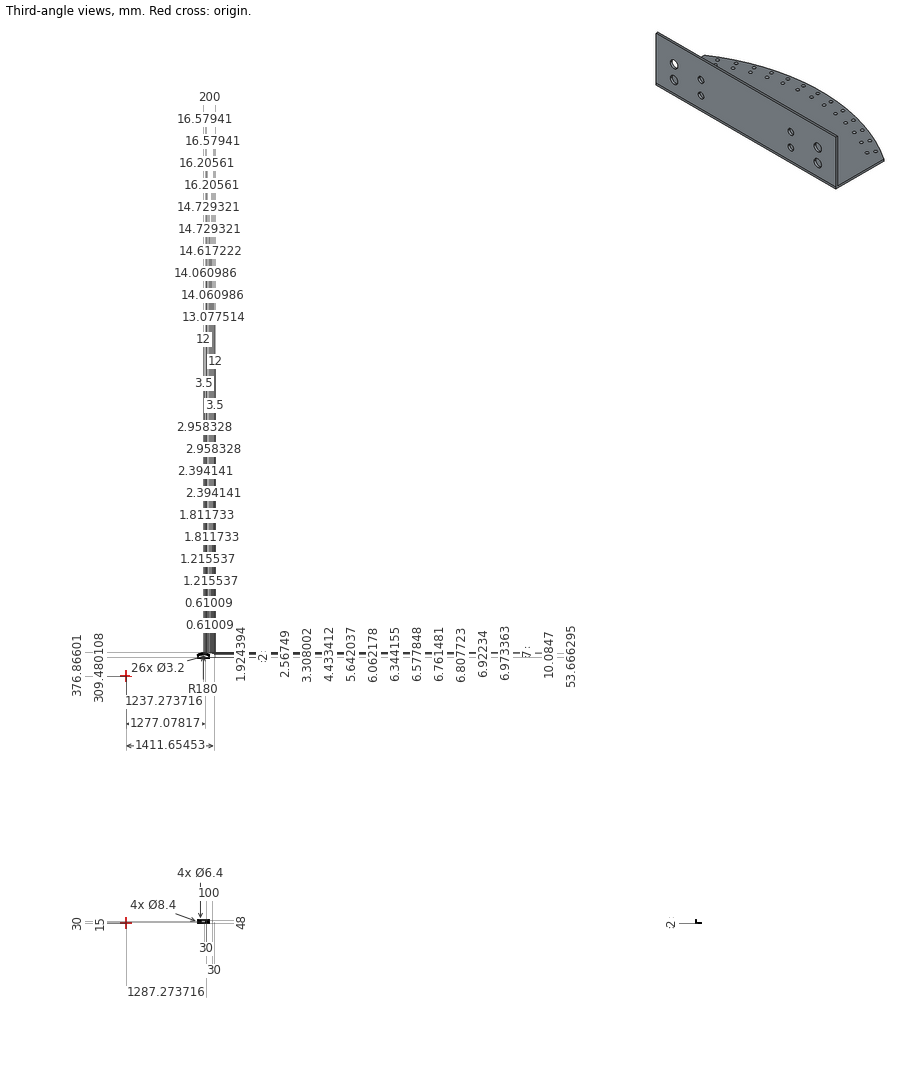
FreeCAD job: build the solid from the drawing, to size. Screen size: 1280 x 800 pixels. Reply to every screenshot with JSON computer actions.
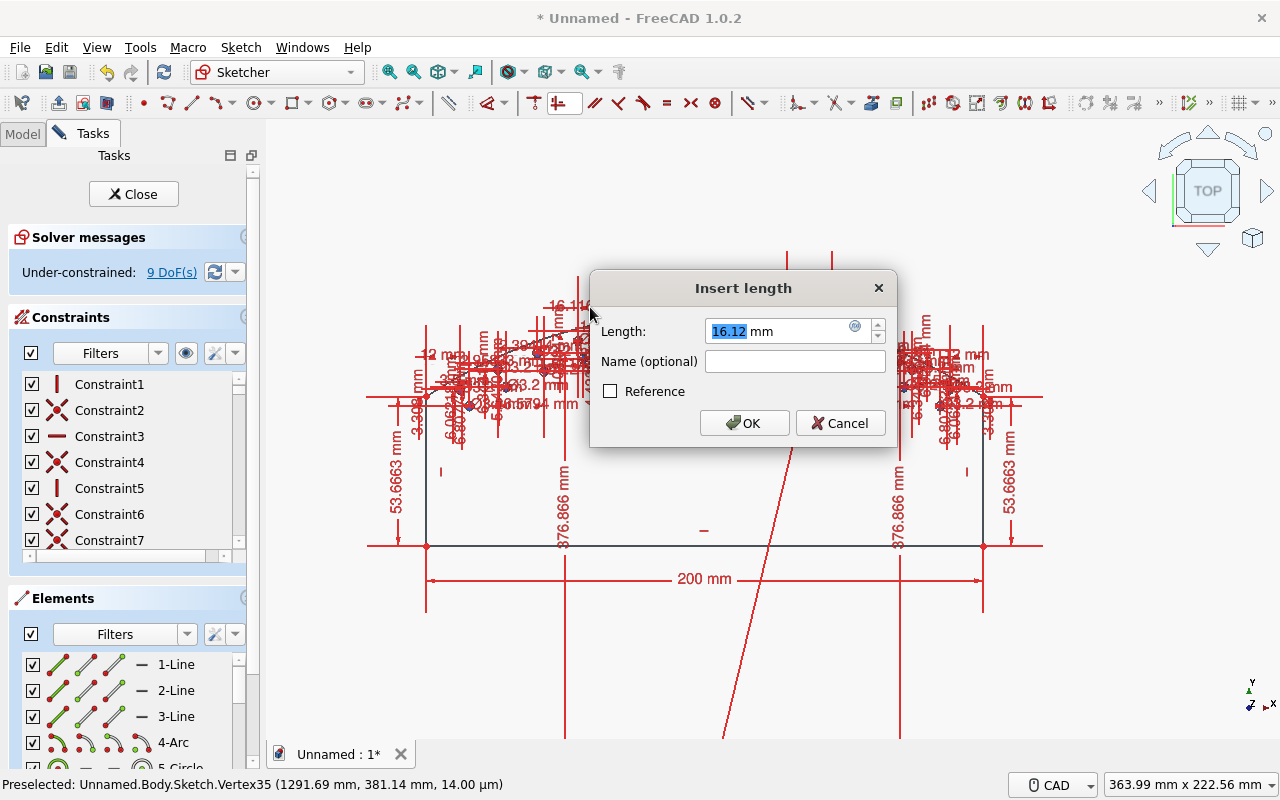
{"action": "type", "text": "16.20561"}
{"action": "key", "text": "Return"}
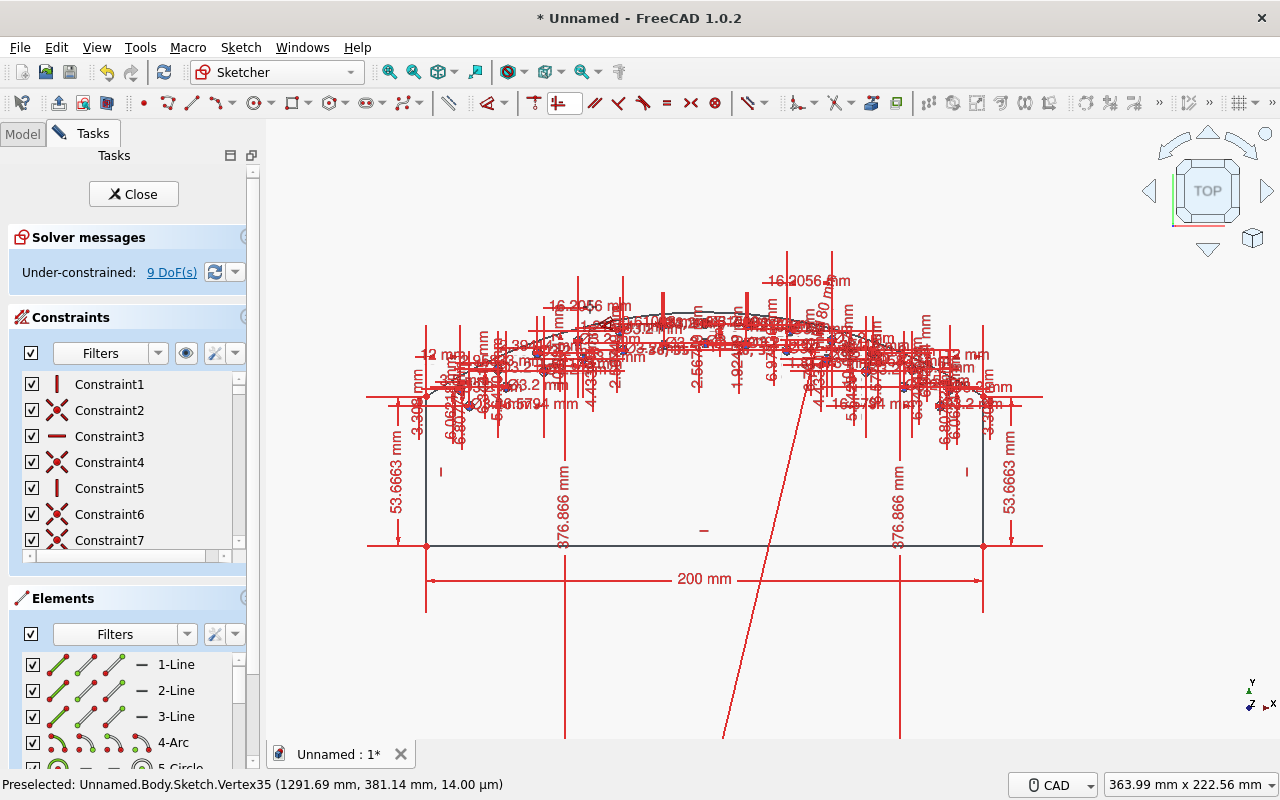
{"action": "scroll", "coordinate": [583, 359], "scroll_direction": "up", "scroll_amount": 4}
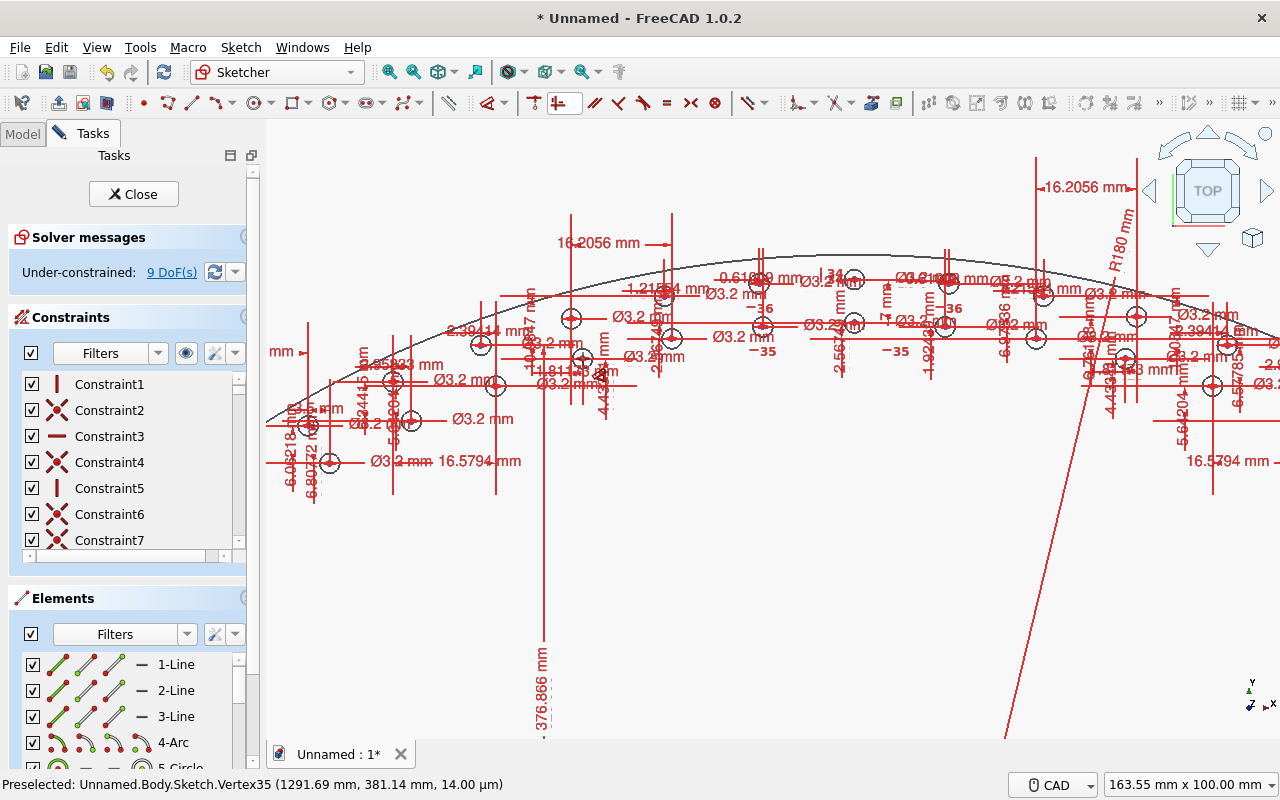
{"action": "left_click", "coordinate": [583, 359]}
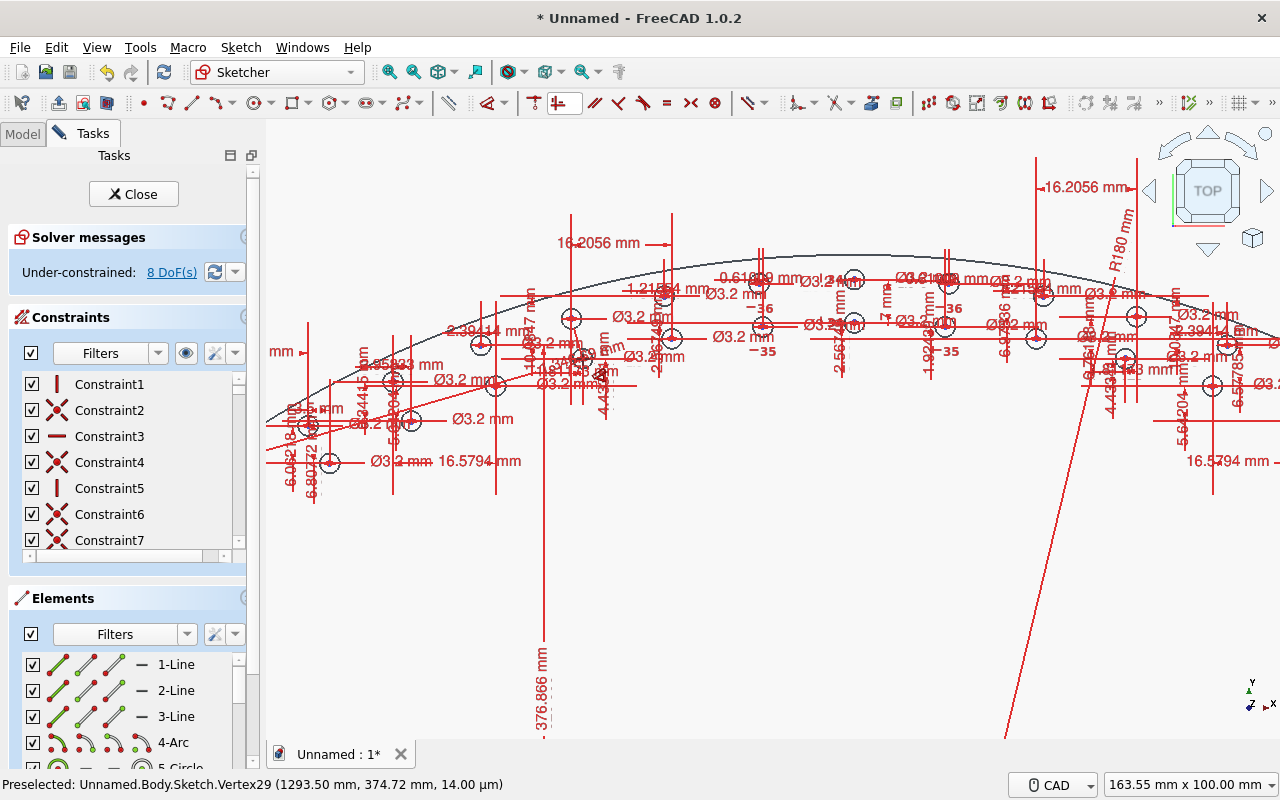
{"action": "left_click", "coordinate": [571, 319]}
{"action": "left_click", "coordinate": [417, 325]}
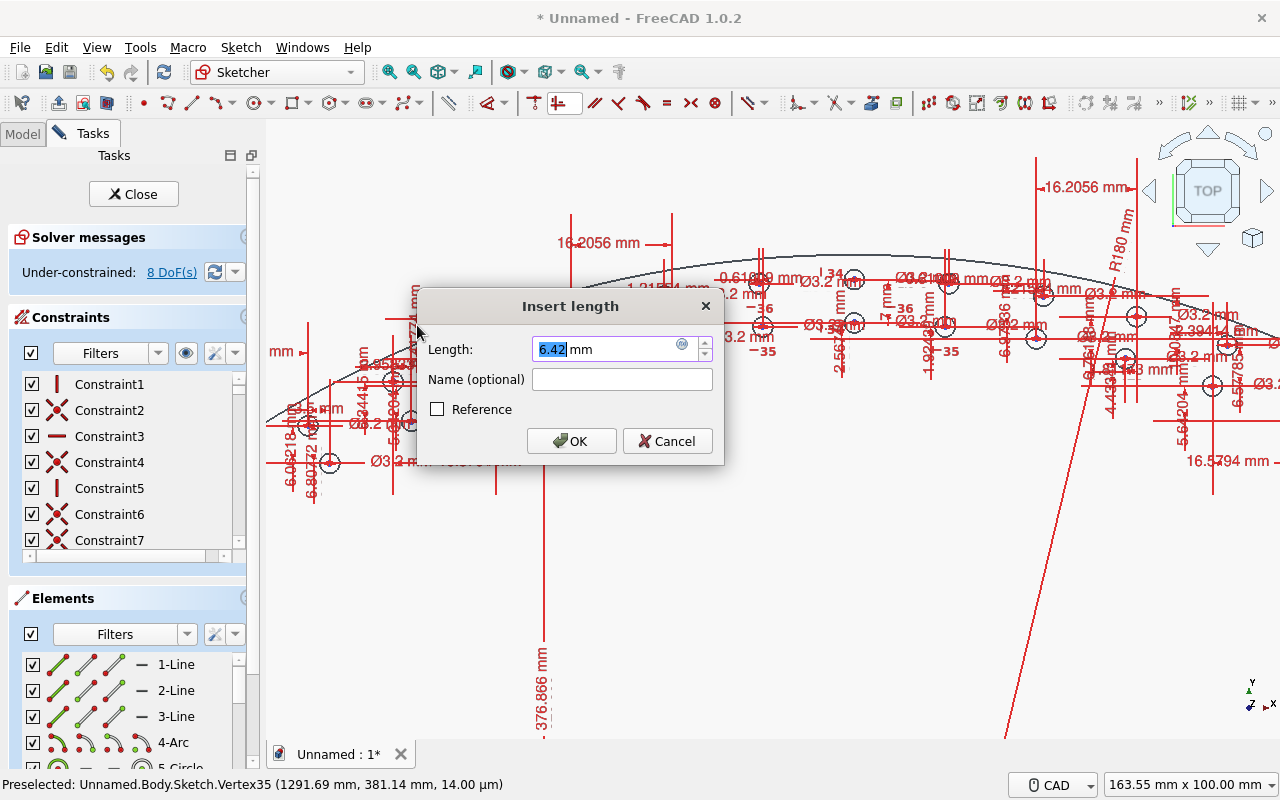
{"action": "type", "text": "6.761481"}
{"action": "key", "text": "Return"}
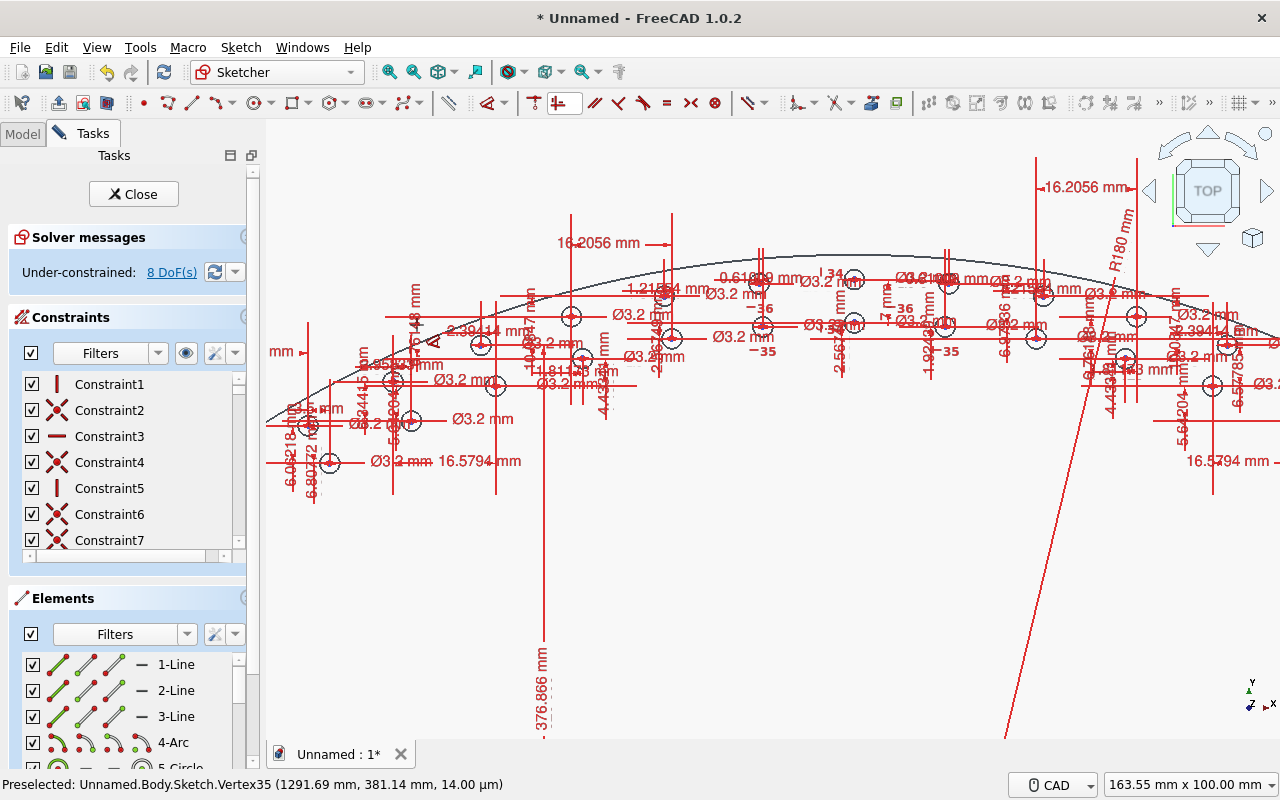
{"action": "scroll", "coordinate": [582, 359], "scroll_direction": "down", "scroll_amount": 4}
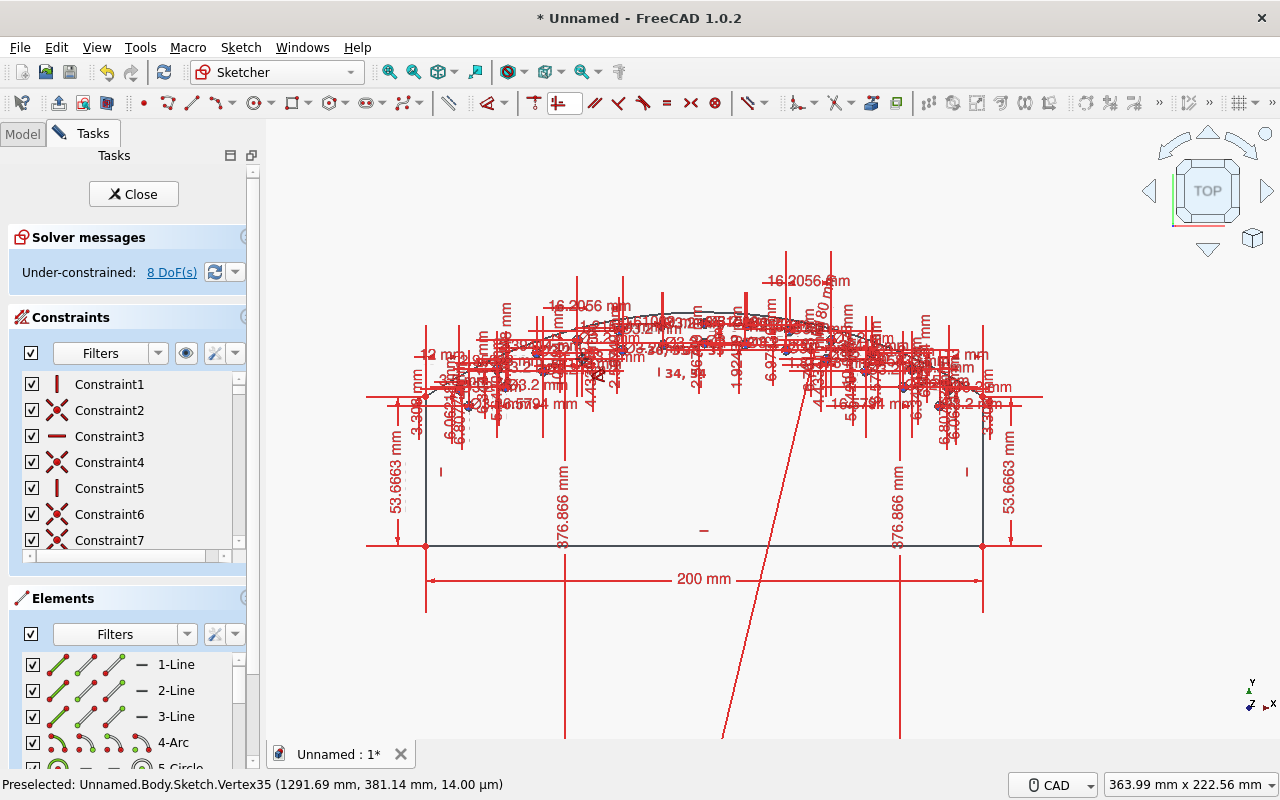
{"action": "left_click", "coordinate": [912, 369]}
{"action": "left_click", "coordinate": [387, 335]}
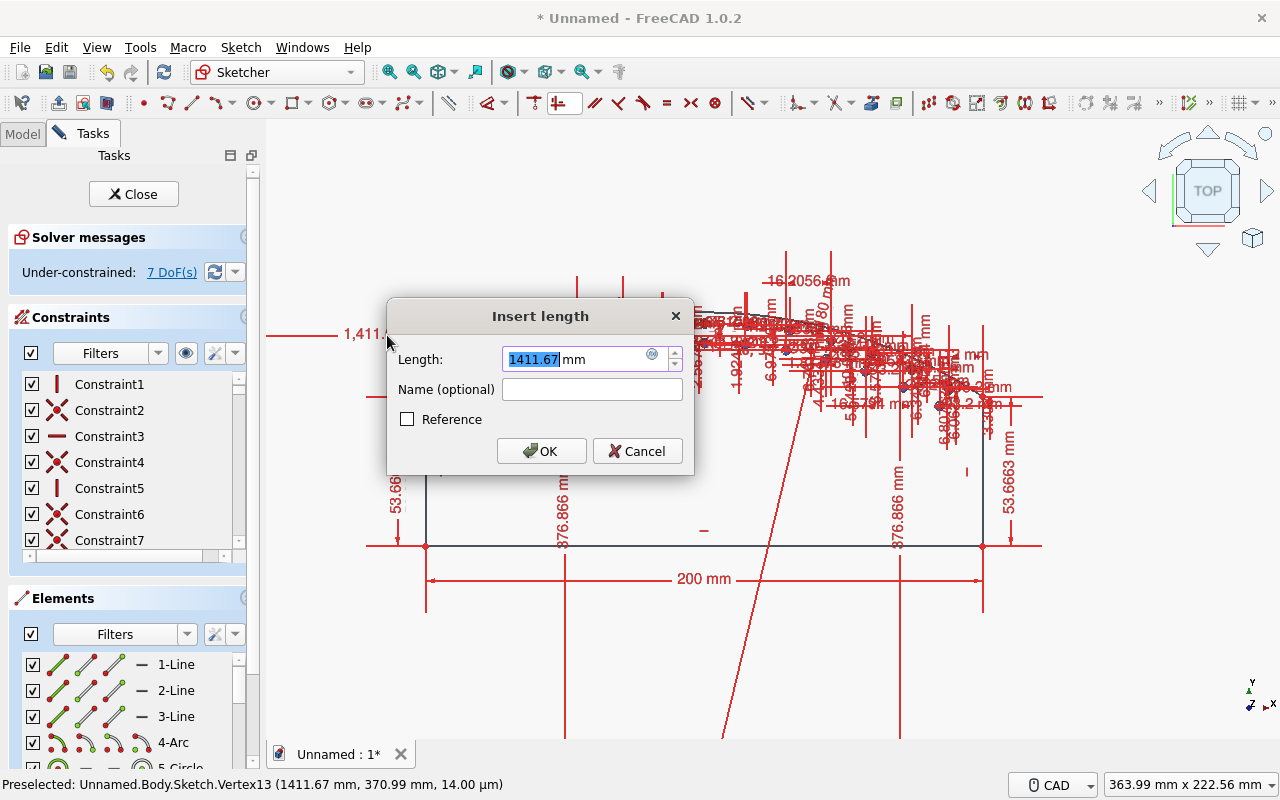
{"action": "type", "text": "1411.65453"}
{"action": "key", "text": "Return"}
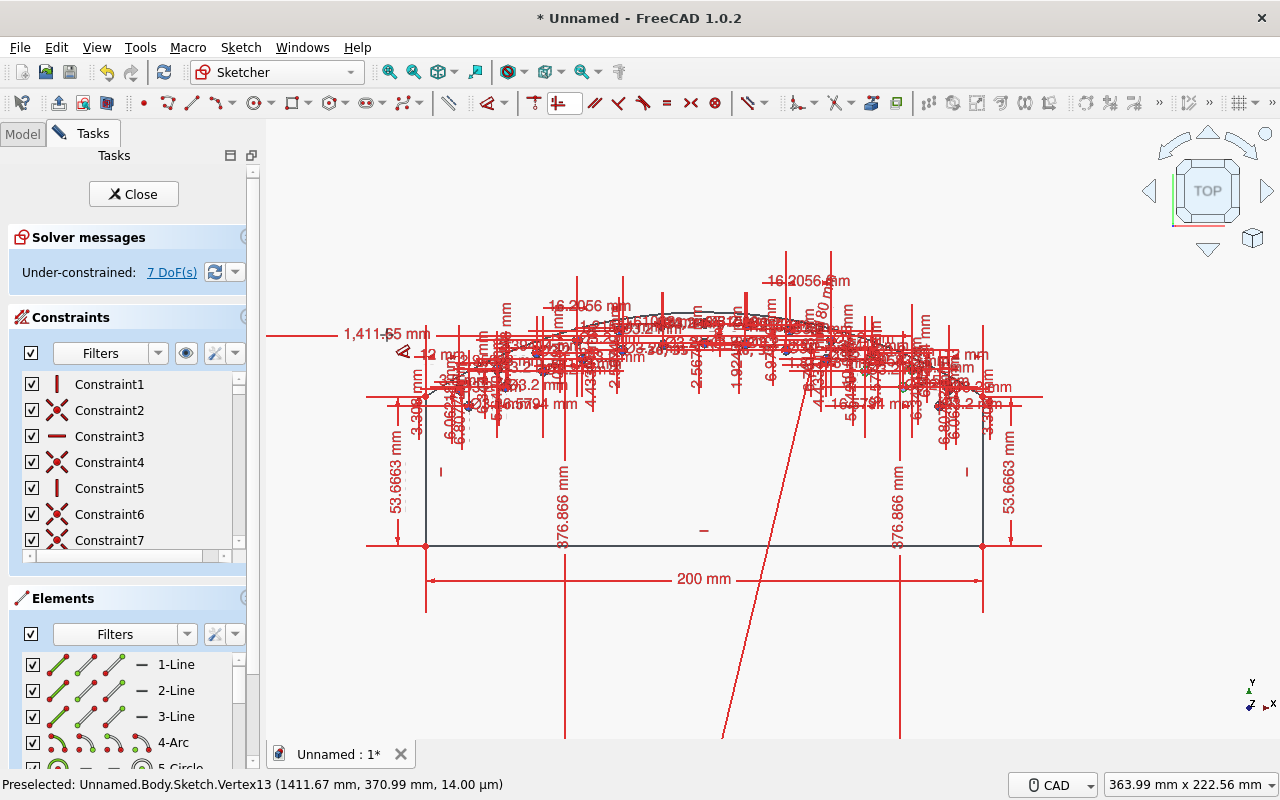
{"action": "left_click", "coordinate": [537, 353]}
{"action": "left_click", "coordinate": [471, 319]}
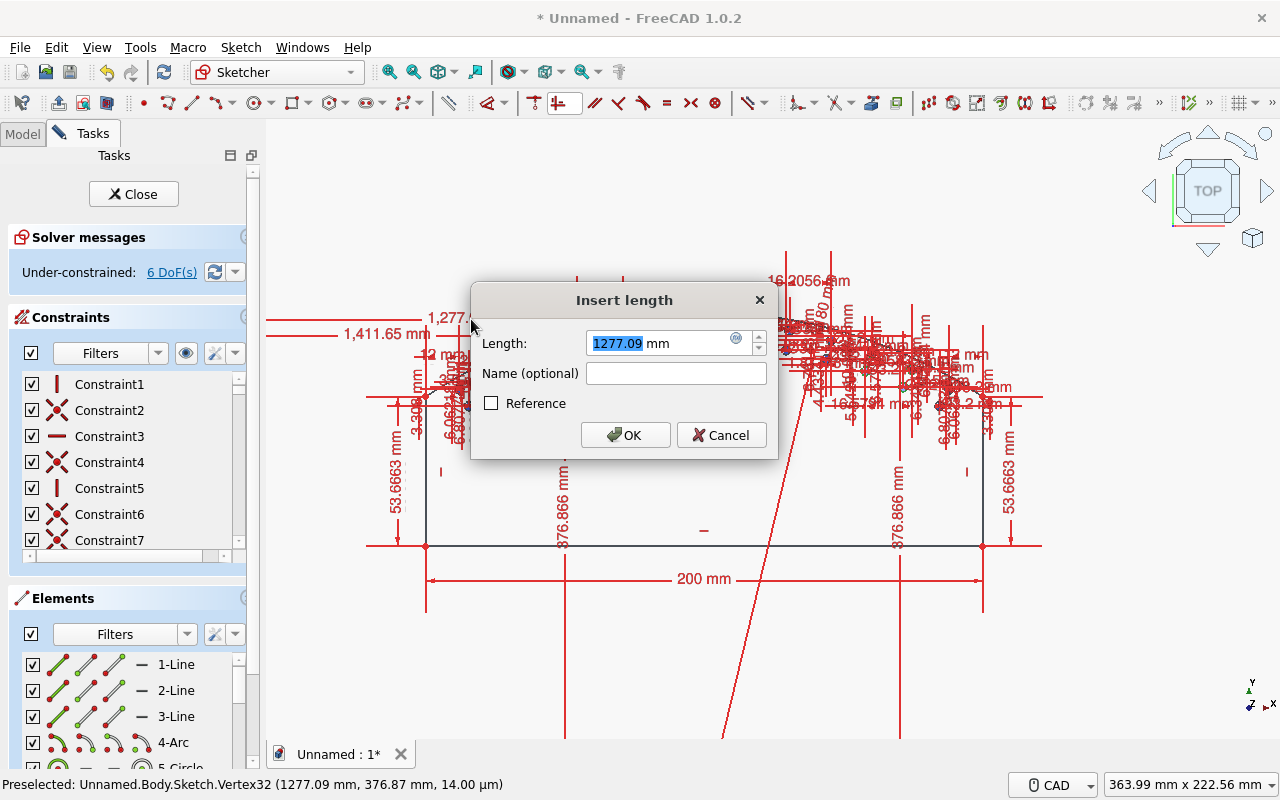
{"action": "type", "text": "1277.07817"}
{"action": "key", "text": "Return"}